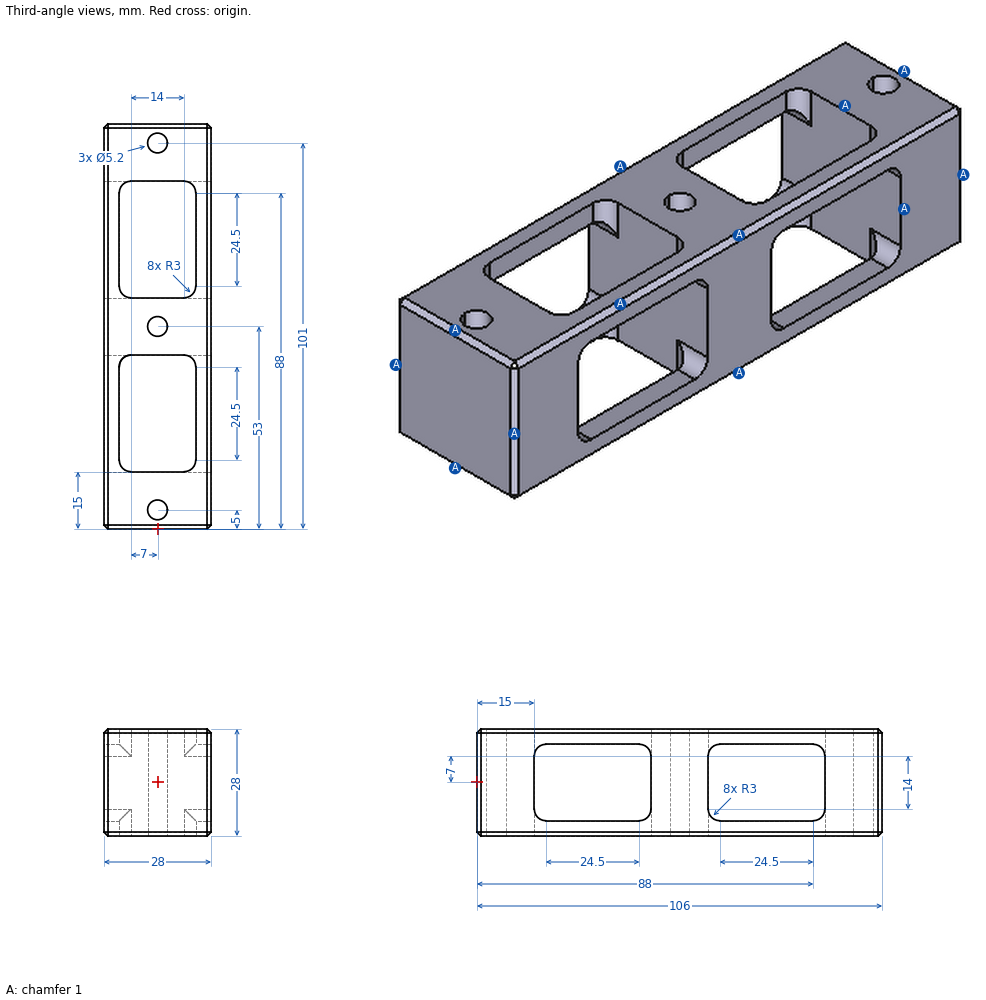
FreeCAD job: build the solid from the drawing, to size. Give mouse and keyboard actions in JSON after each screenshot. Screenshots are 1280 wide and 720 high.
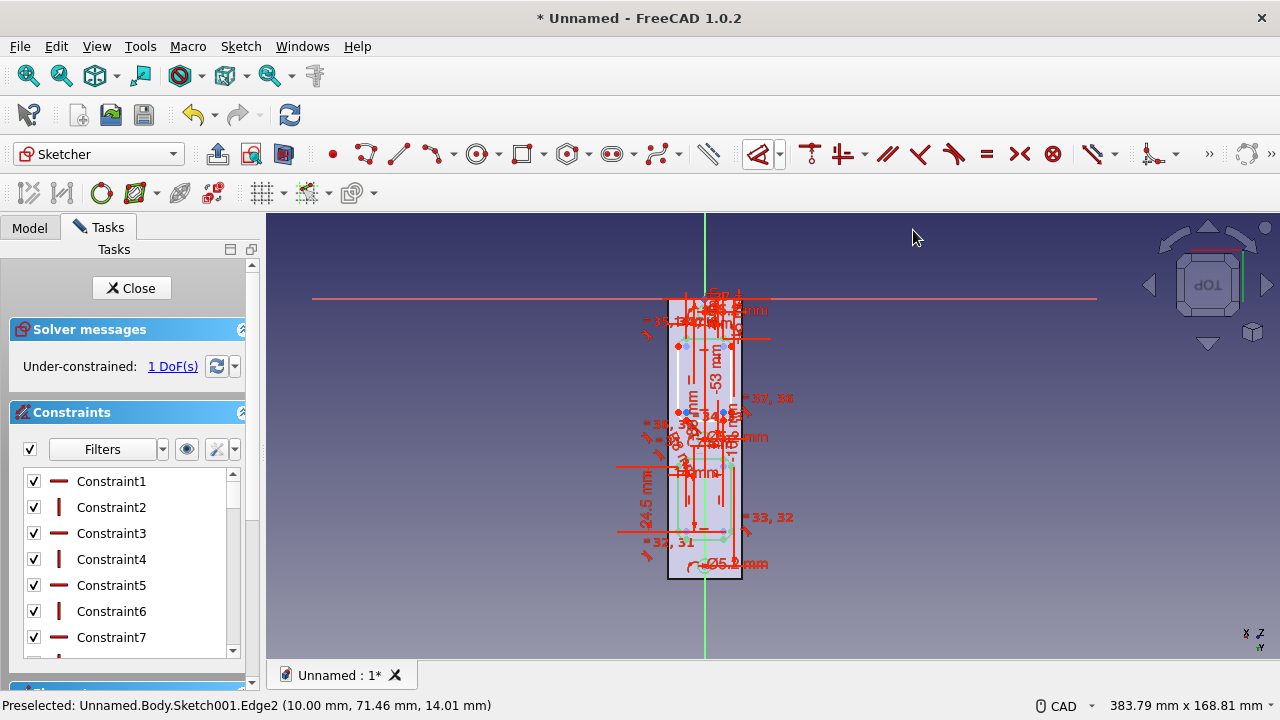
{"action": "left_click", "coordinate": [678, 367]}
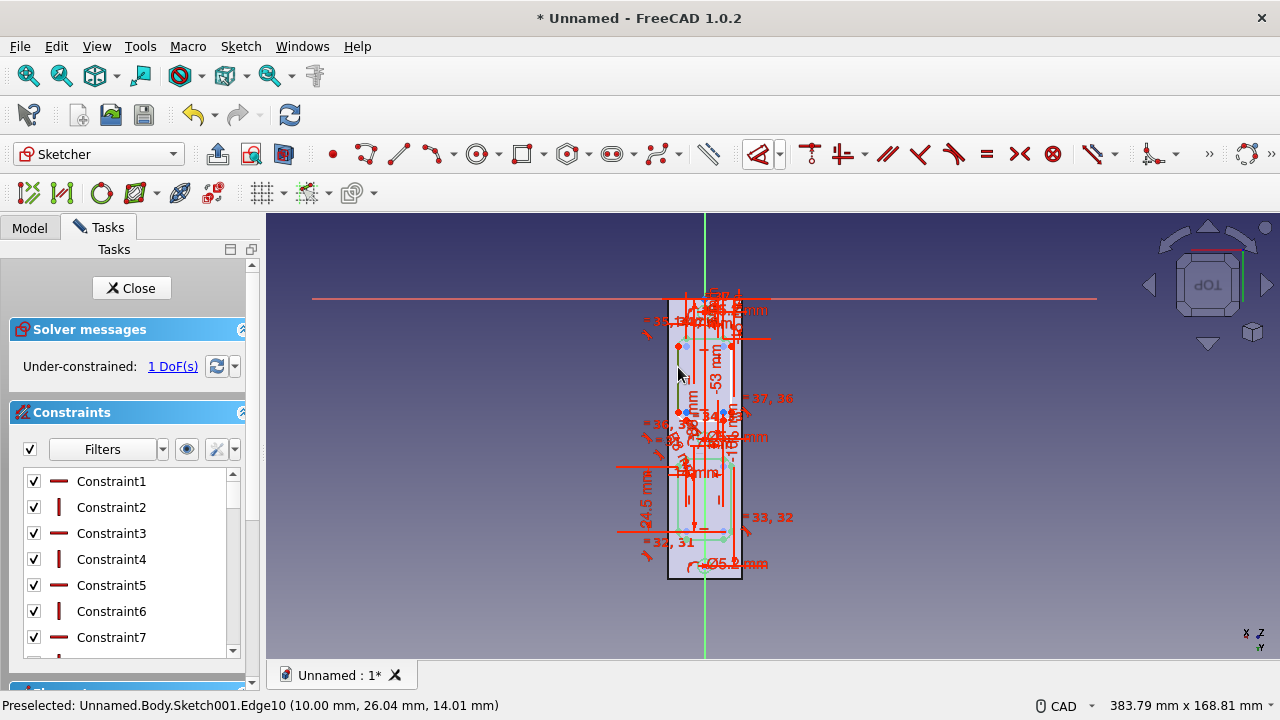
{"action": "key", "text": "i"}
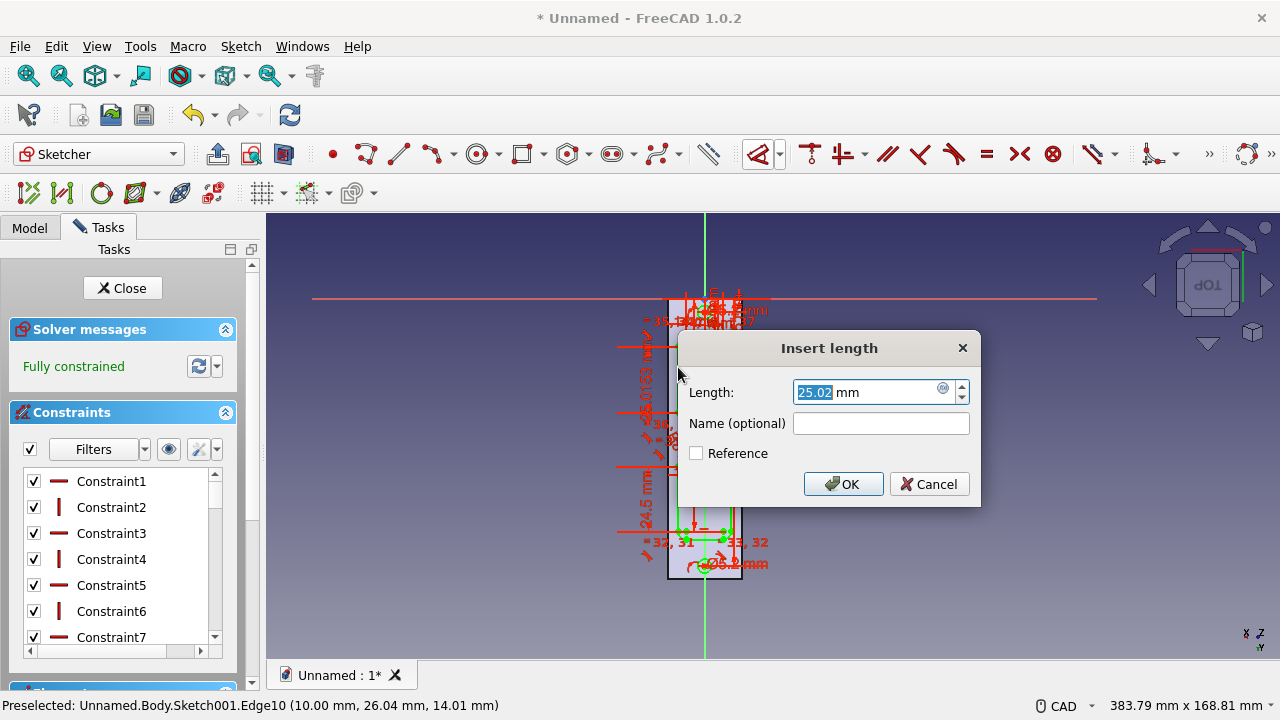
{"action": "type", "text": "24.5"}
{"action": "key", "text": "Return"}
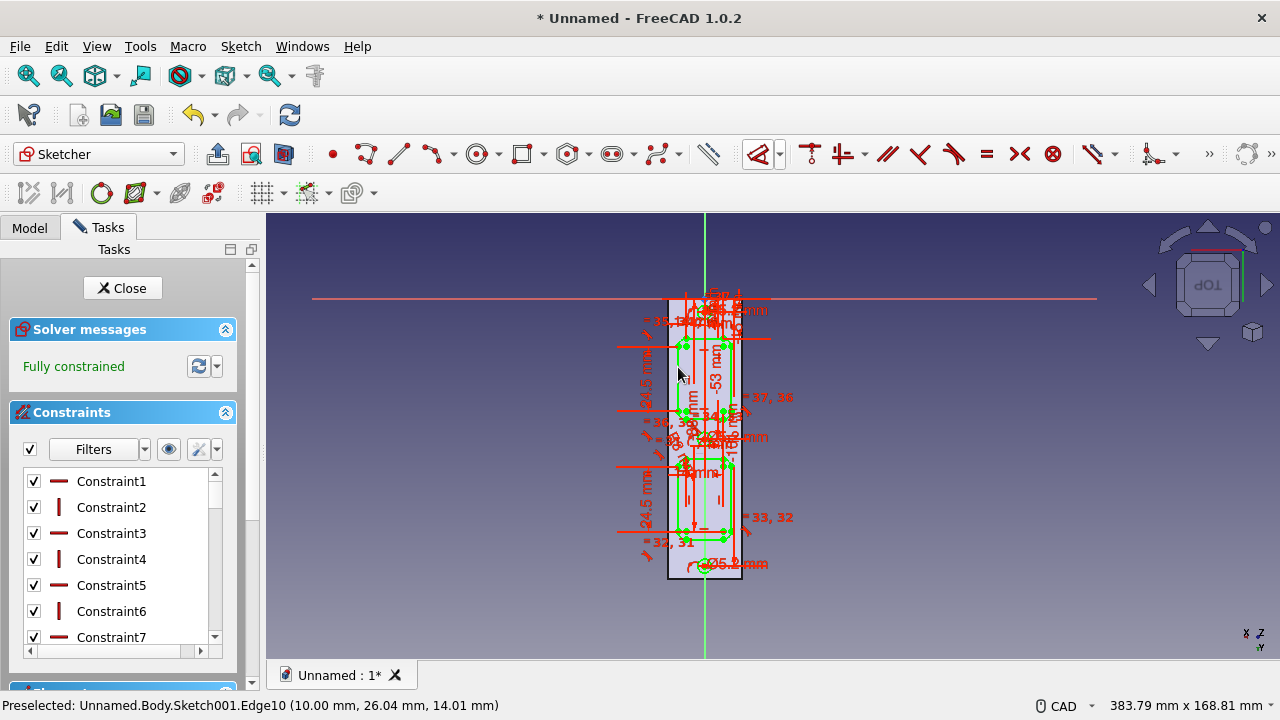
{"action": "left_click", "coordinate": [123, 288]}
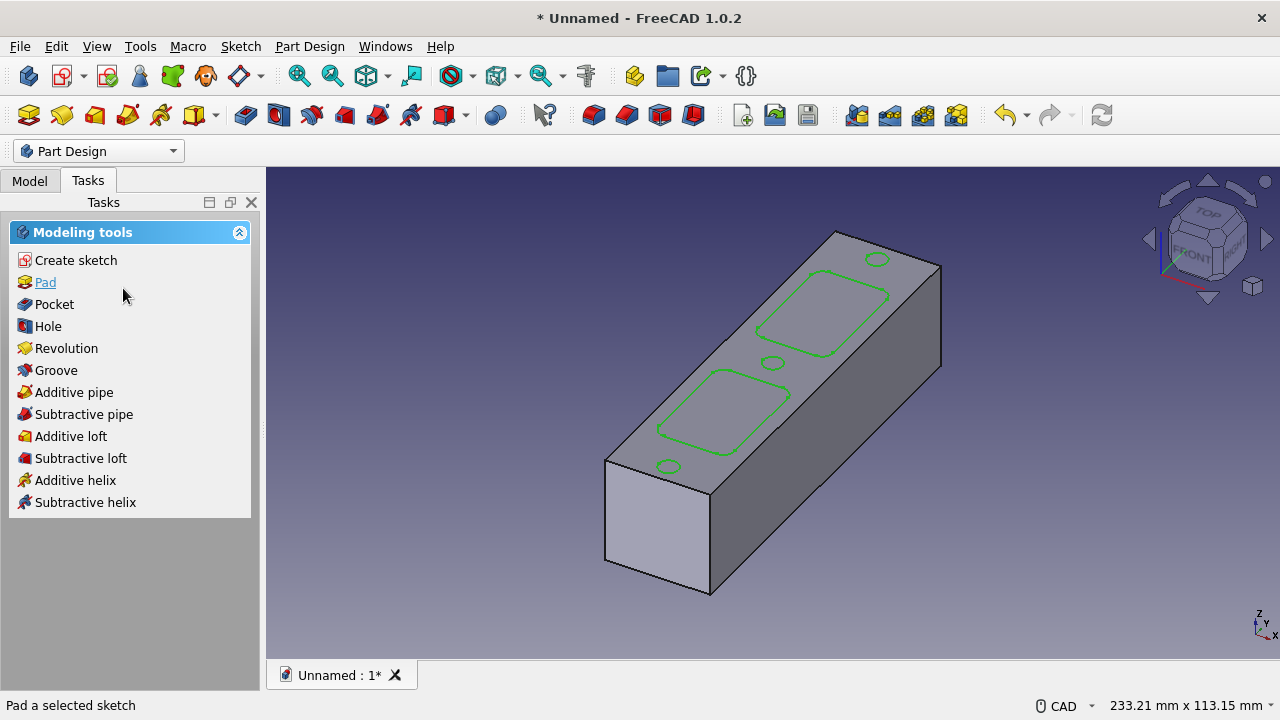
{"action": "left_click", "coordinate": [246, 116]}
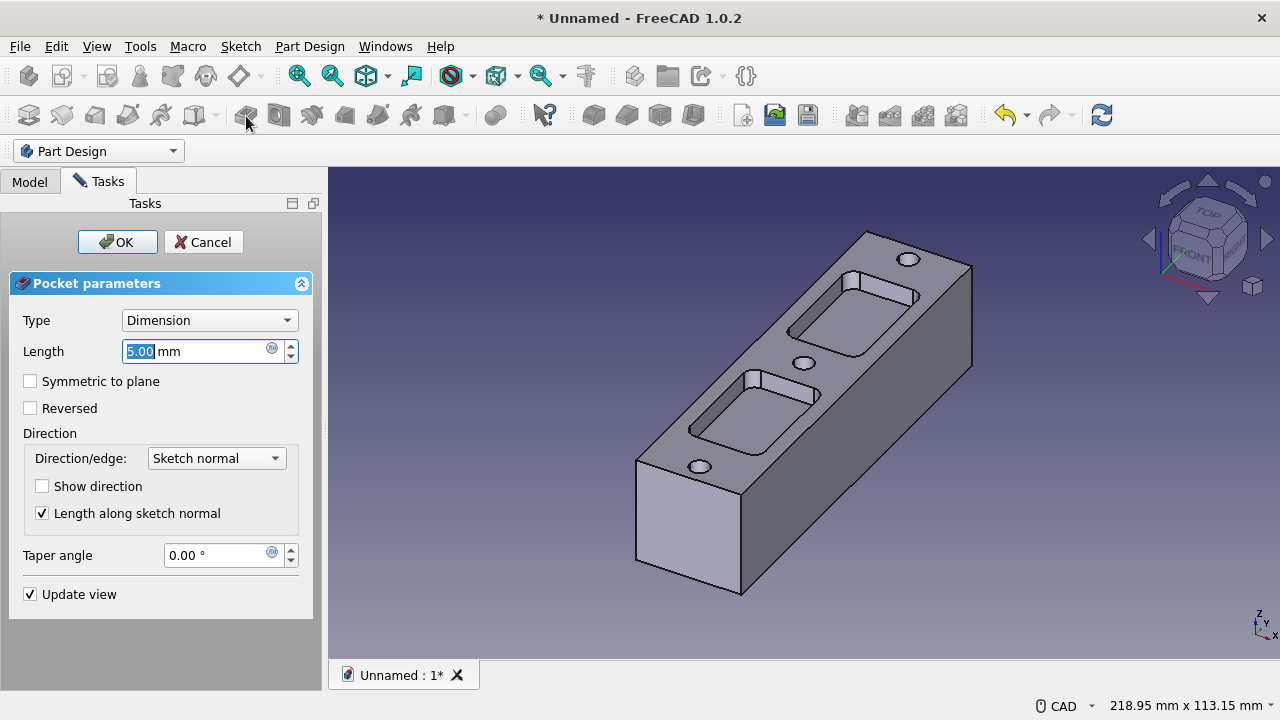
{"action": "left_click", "coordinate": [210, 320]}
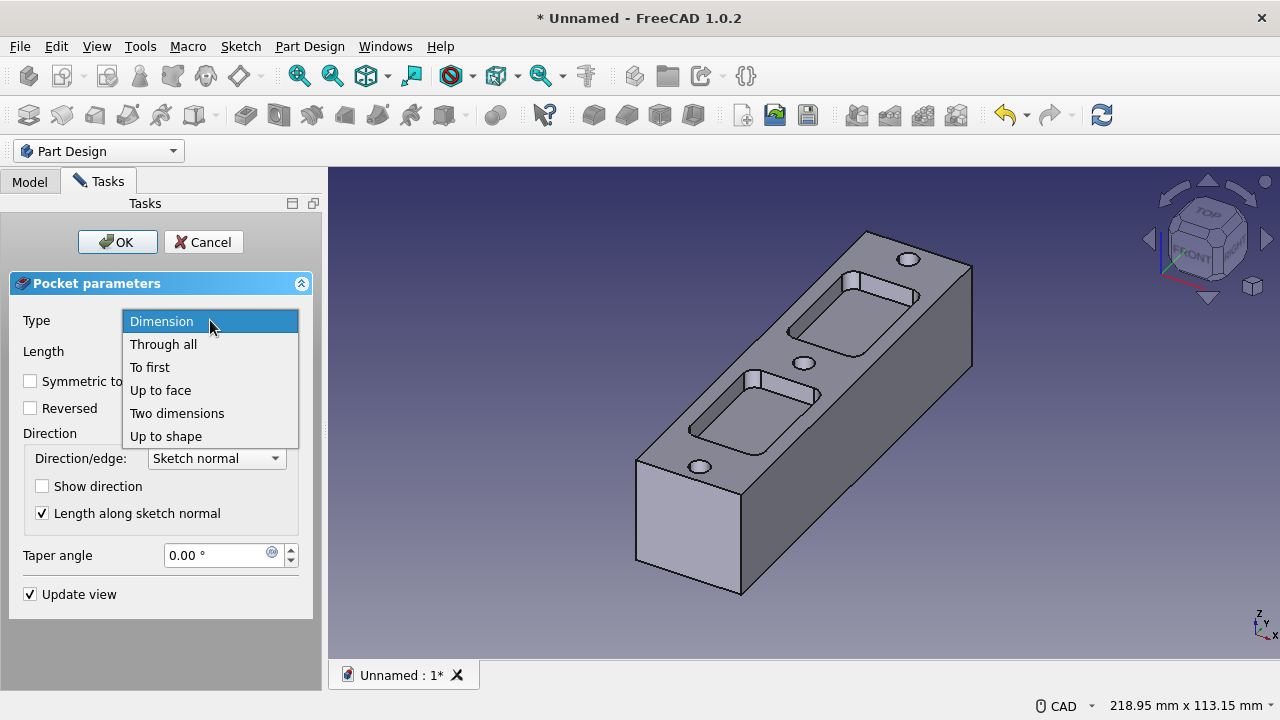
{"action": "left_click", "coordinate": [208, 344]}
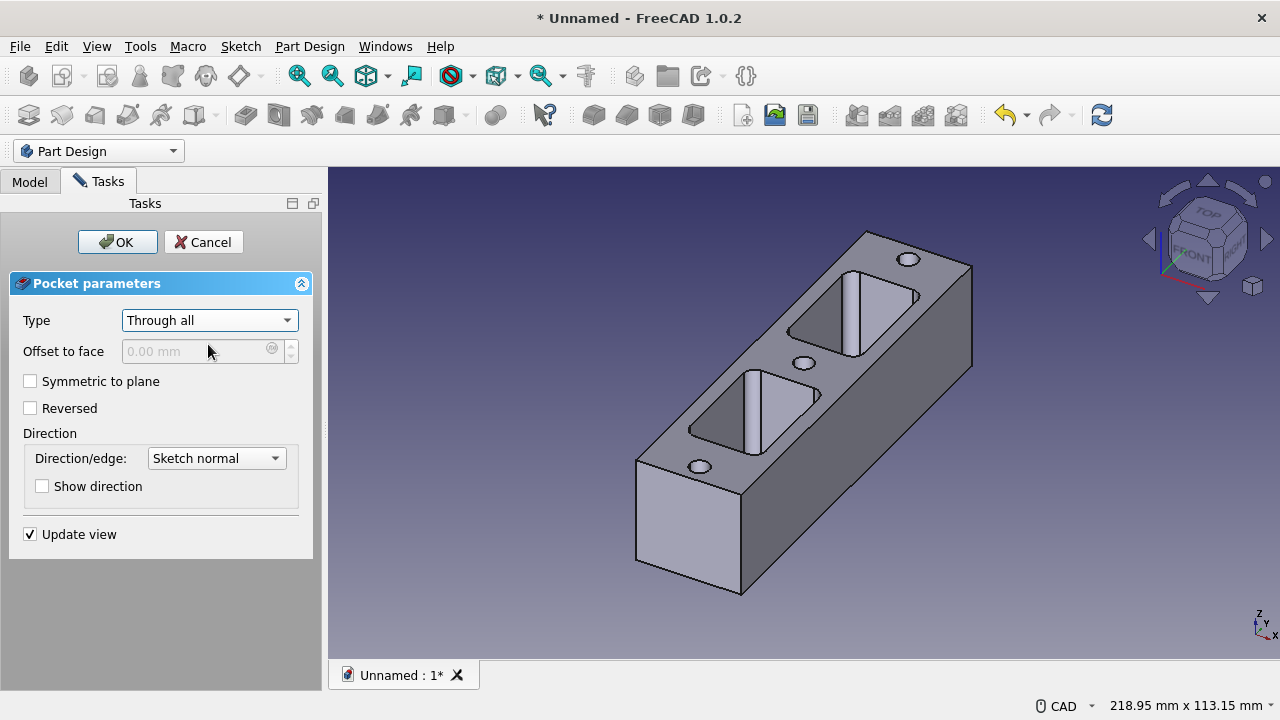
{"action": "left_click", "coordinate": [118, 242]}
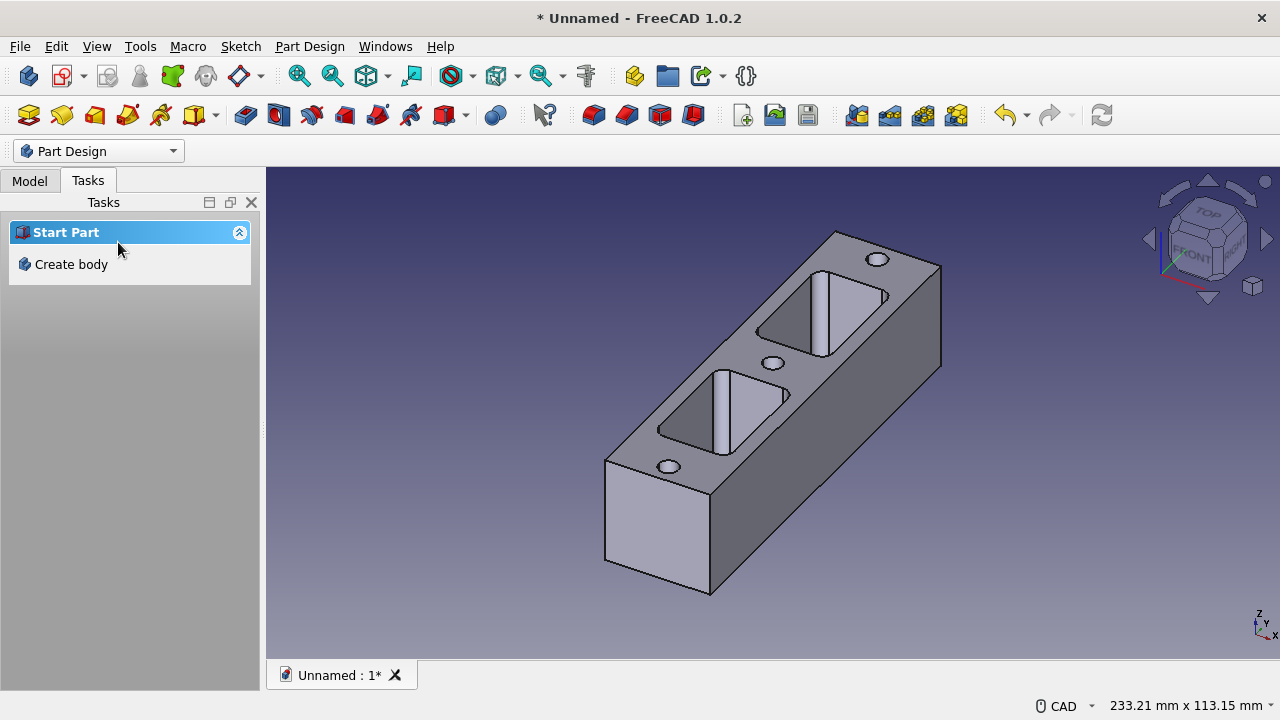
{"action": "left_click", "coordinate": [760, 495]}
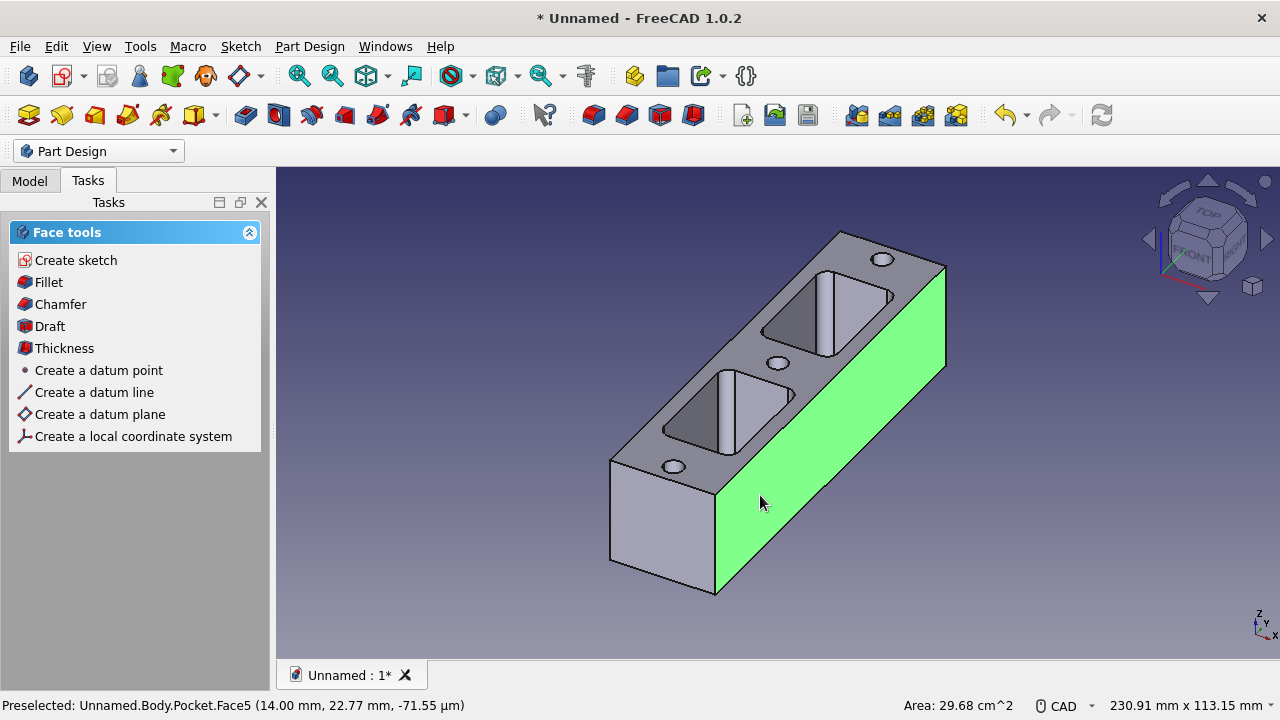
{"action": "left_click", "coordinate": [62, 76]}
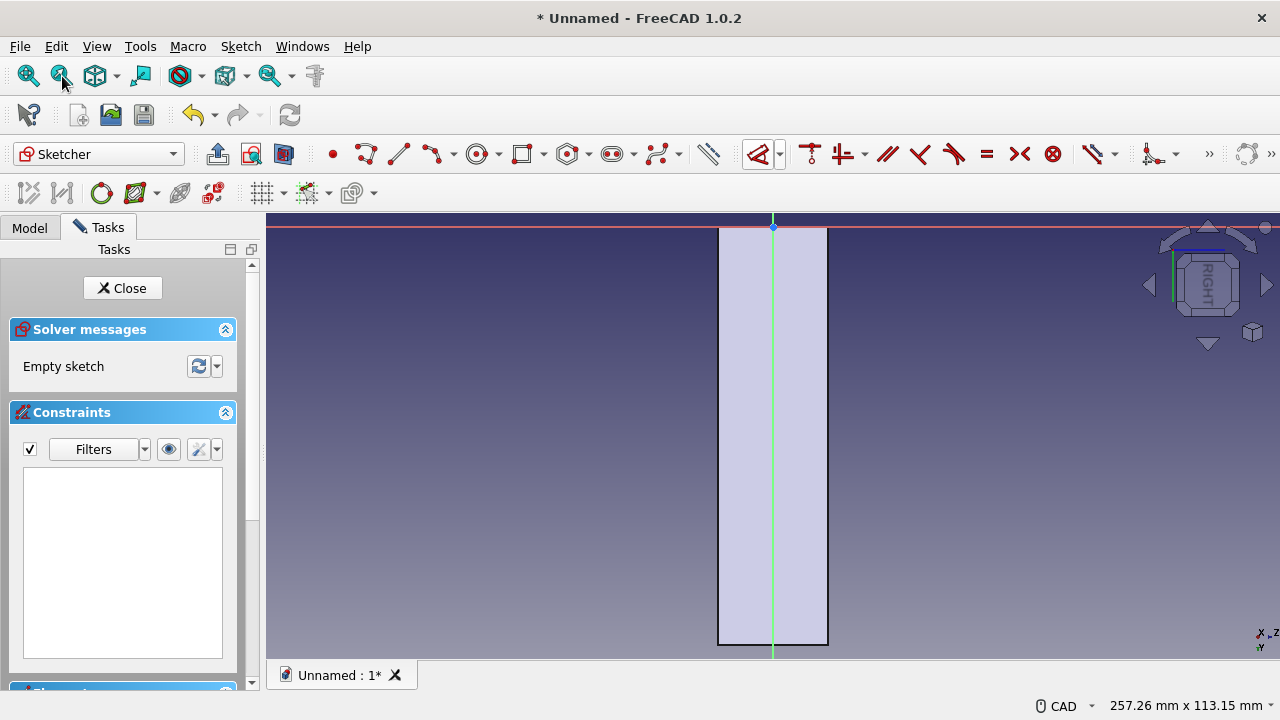
{"action": "scroll", "coordinate": [395, 570], "scroll_direction": "down", "scroll_amount": 1}